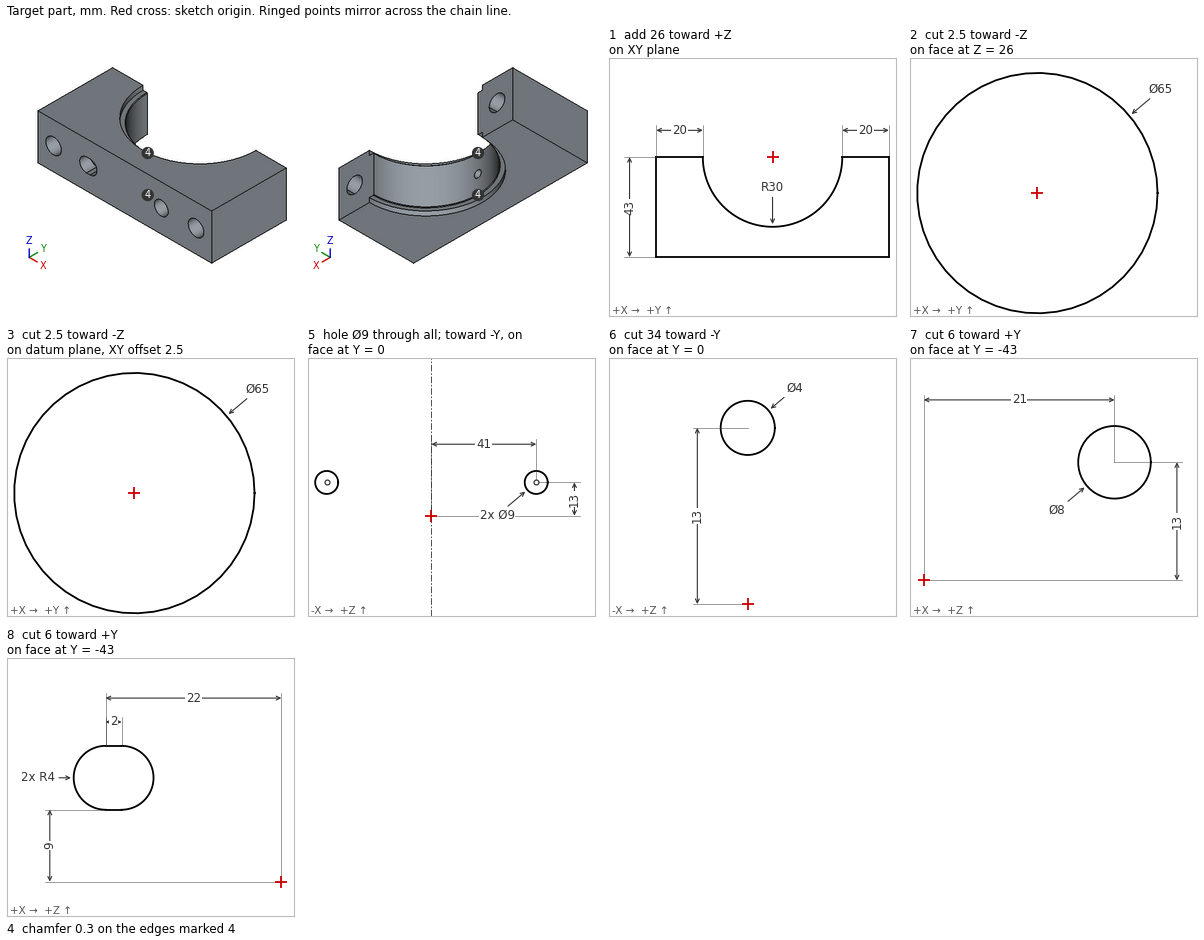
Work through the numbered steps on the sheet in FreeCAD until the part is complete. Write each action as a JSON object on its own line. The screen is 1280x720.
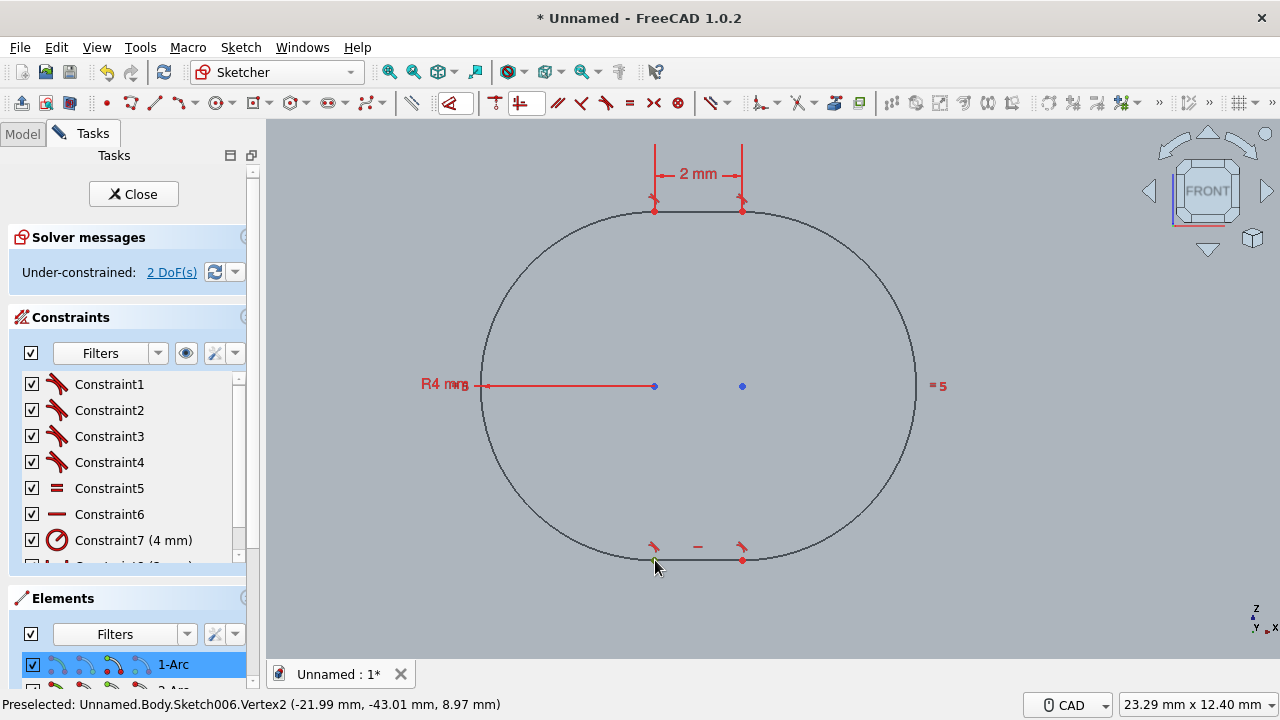
{"action": "left_click", "coordinate": [468, 104]}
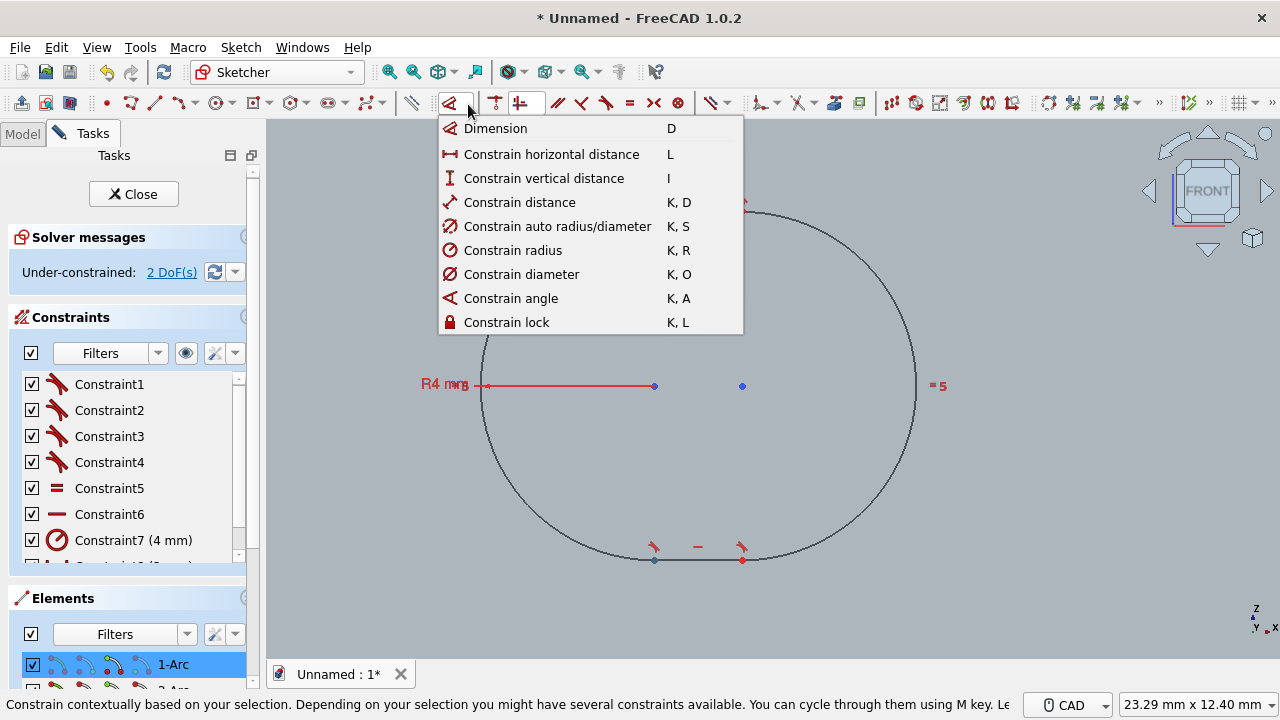
{"action": "left_click", "coordinate": [591, 178]}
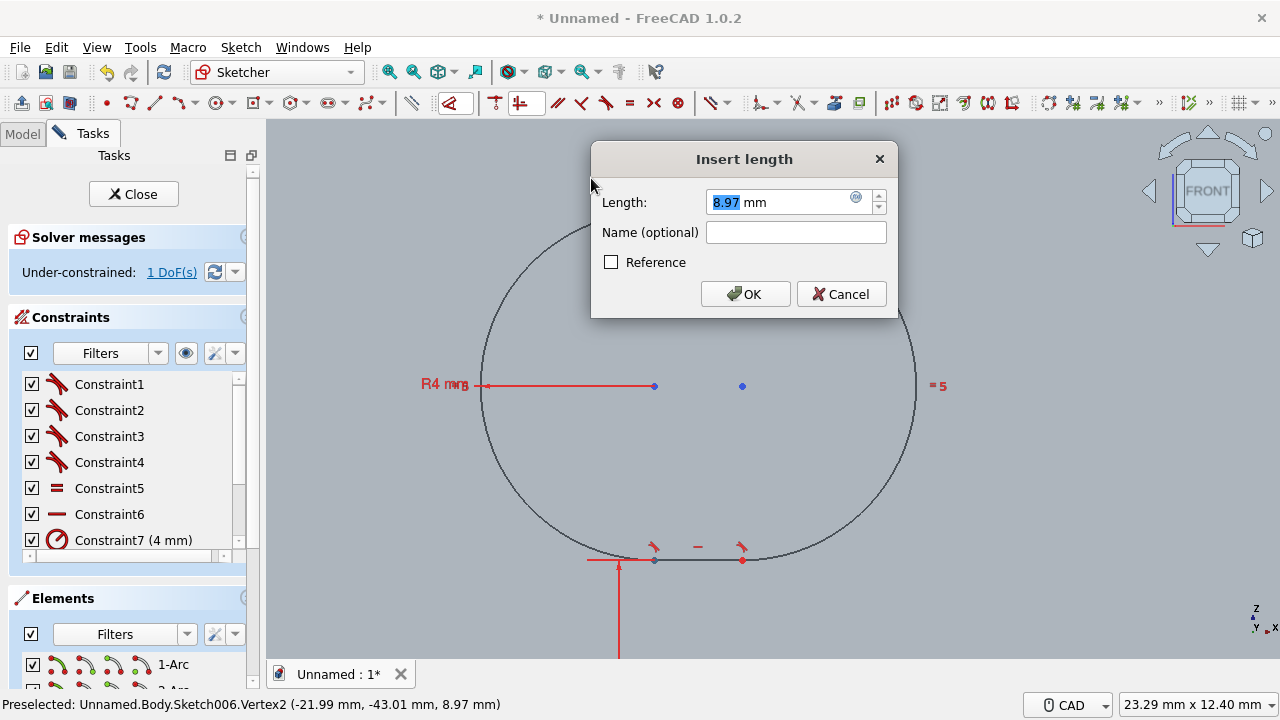
{"action": "type", "text": "9"}
{"action": "key", "text": "Return"}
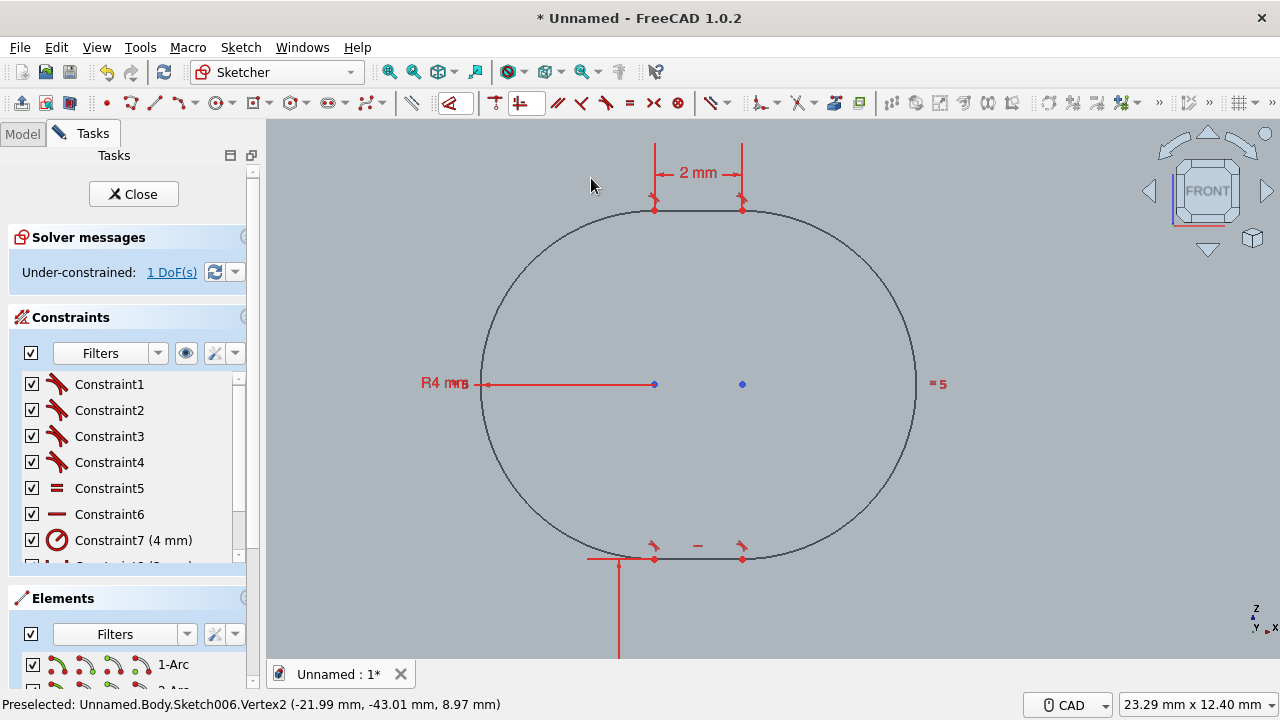
{"action": "left_click", "coordinate": [655, 211]}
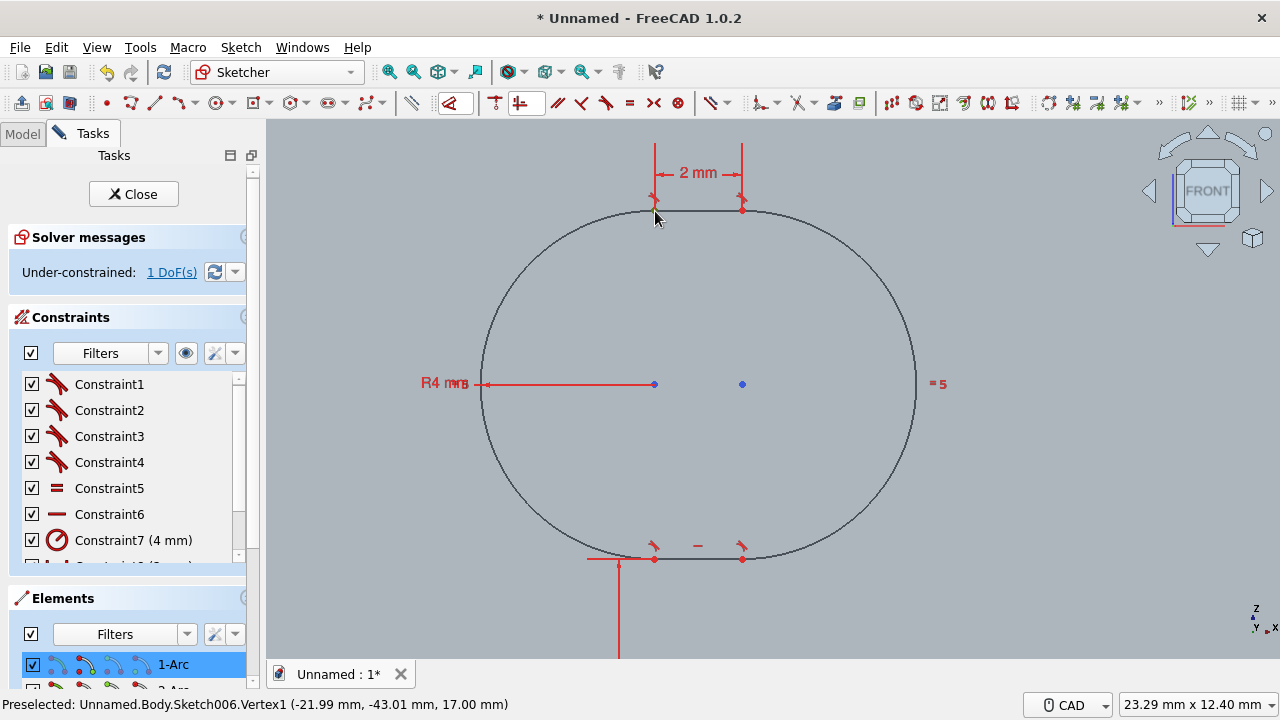
{"action": "left_click", "coordinate": [468, 104]}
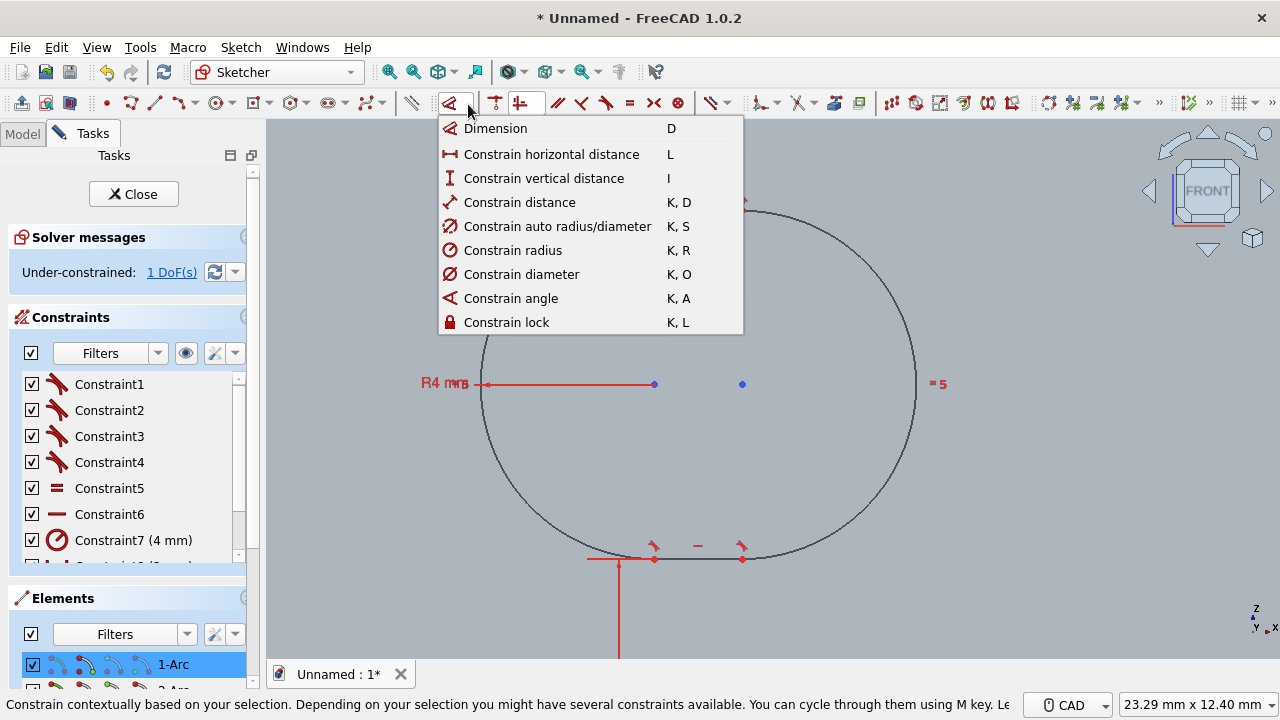
{"action": "left_click", "coordinate": [591, 154]}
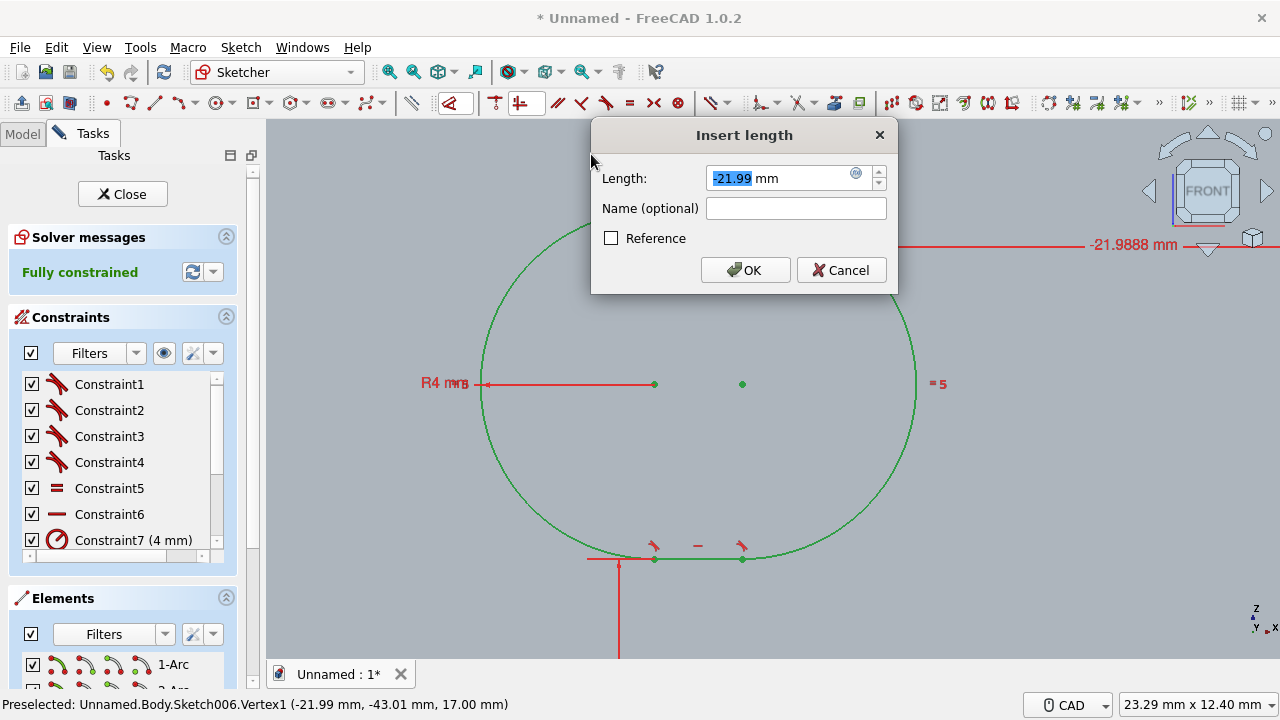
{"action": "type", "text": "-22"}
{"action": "key", "text": "Return"}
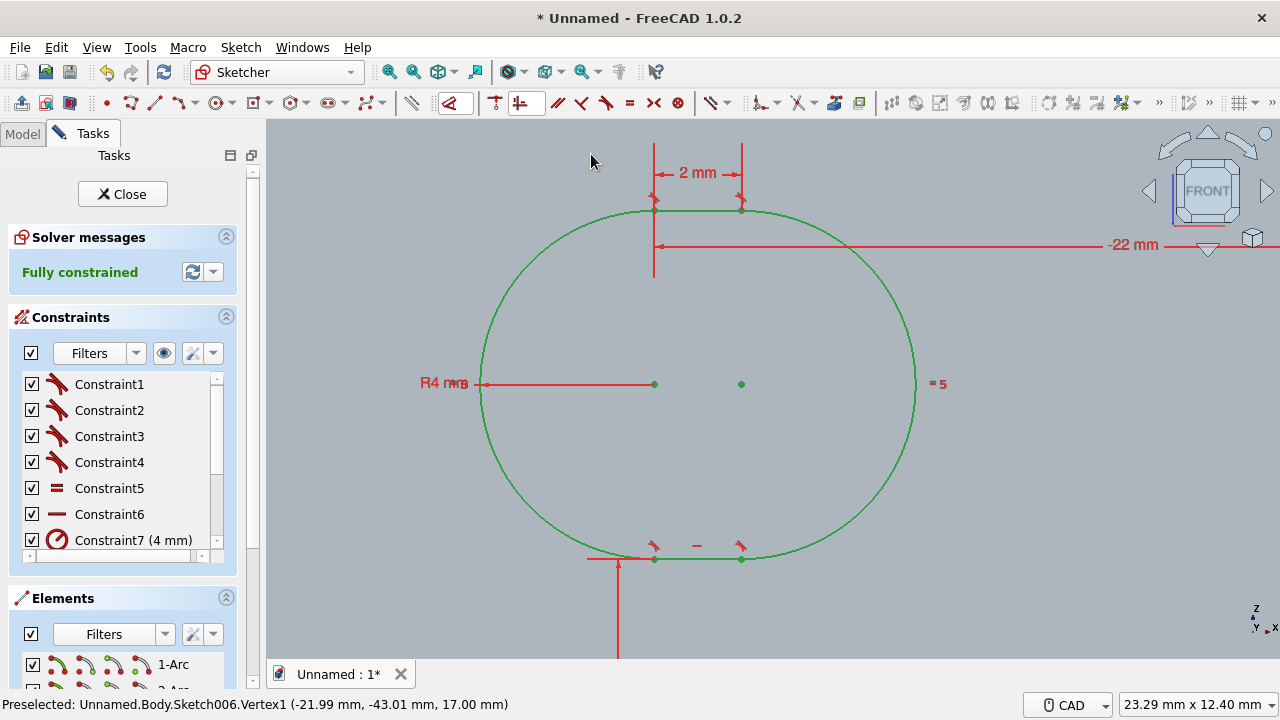
{"action": "left_click", "coordinate": [123, 194]}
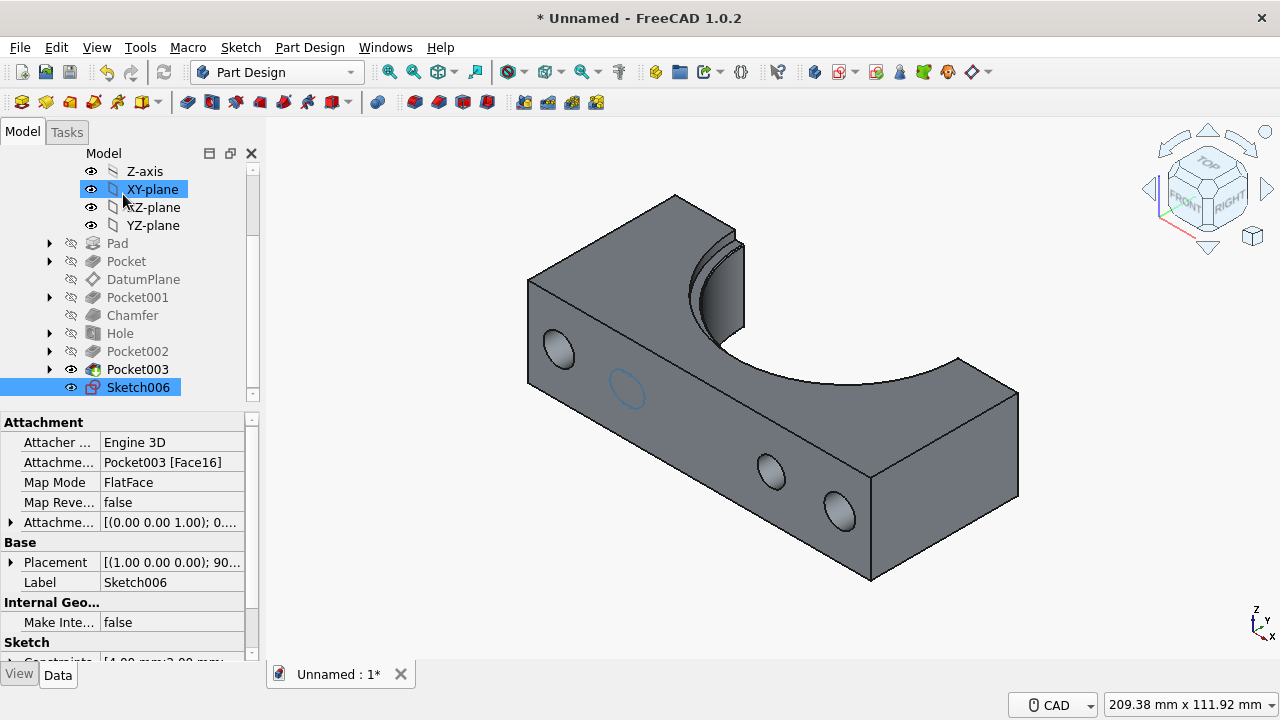
{"action": "left_click", "coordinate": [188, 102]}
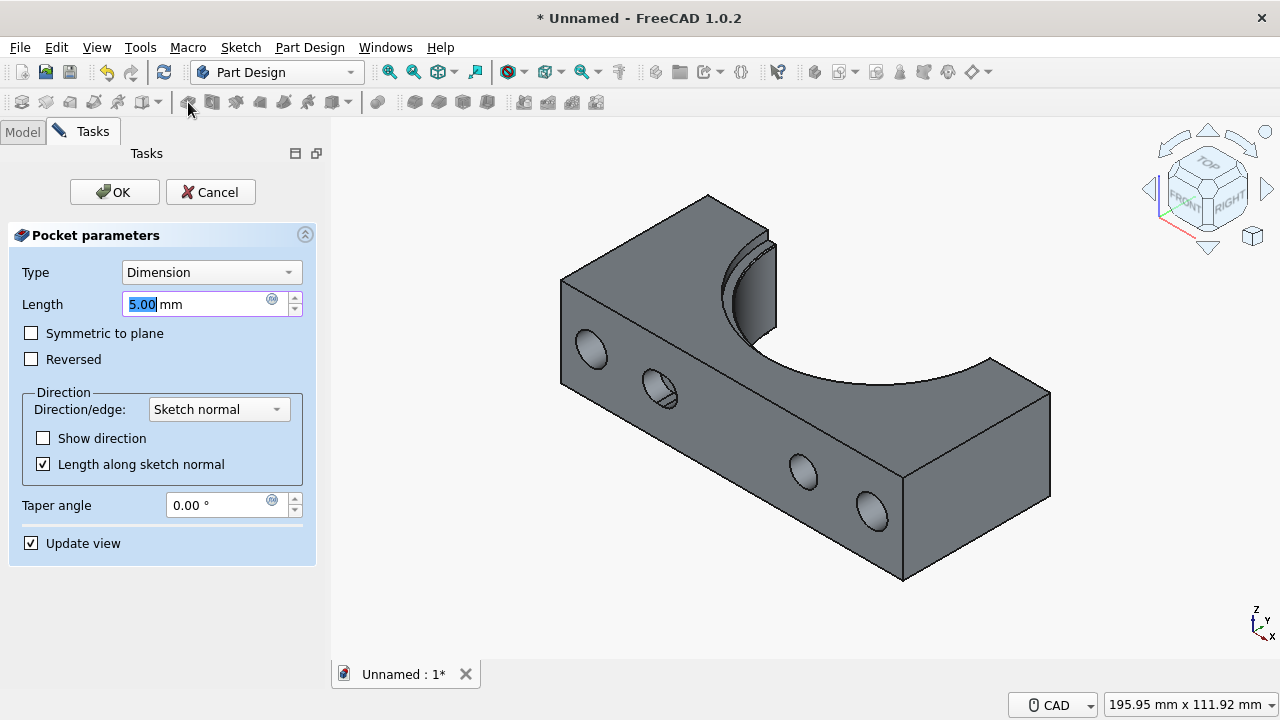
{"action": "type", "text": "6"}
{"action": "key", "text": "Tab"}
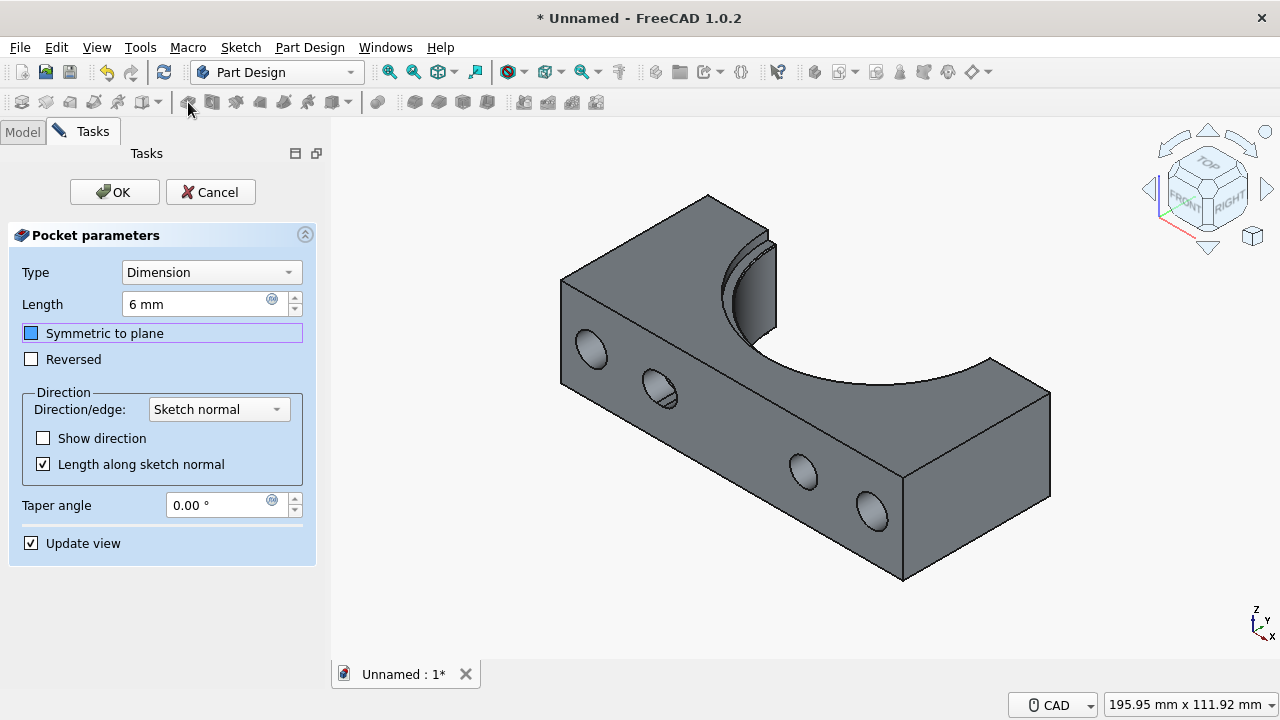
{"action": "left_click", "coordinate": [115, 192]}